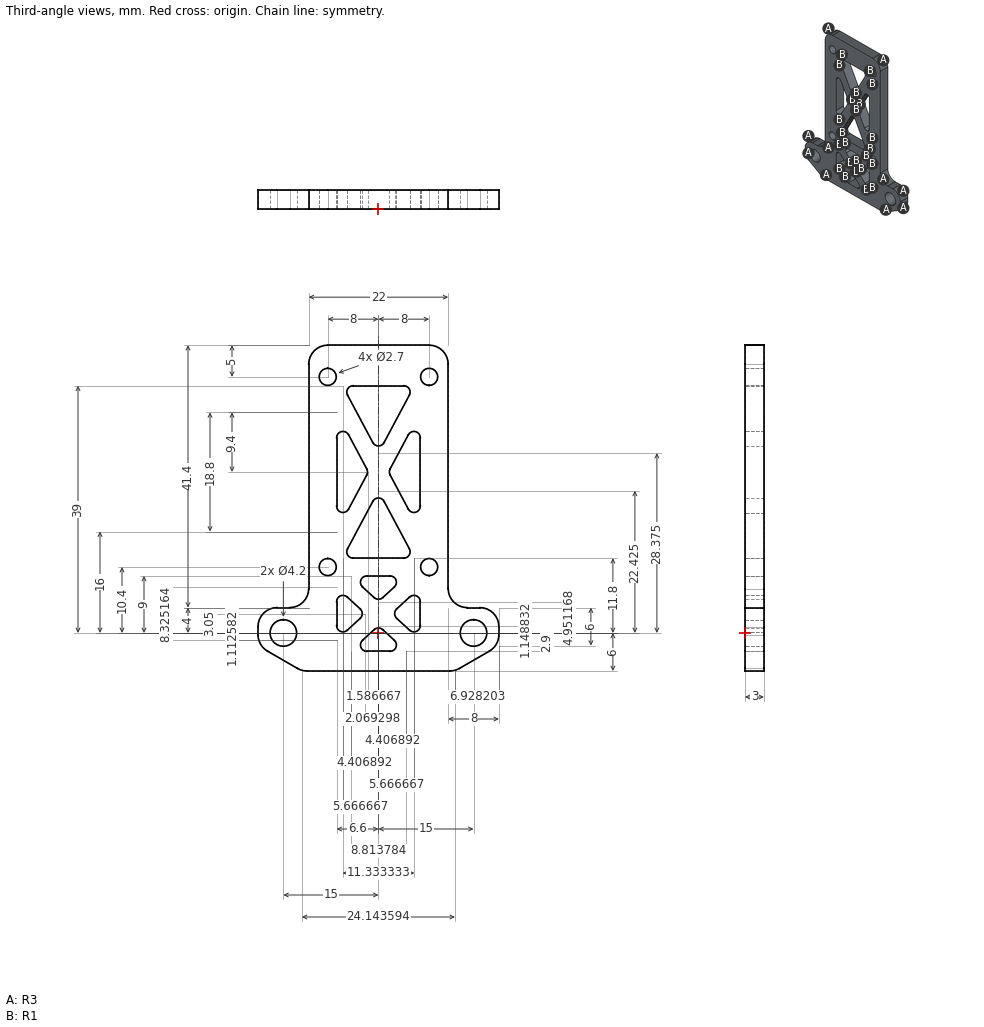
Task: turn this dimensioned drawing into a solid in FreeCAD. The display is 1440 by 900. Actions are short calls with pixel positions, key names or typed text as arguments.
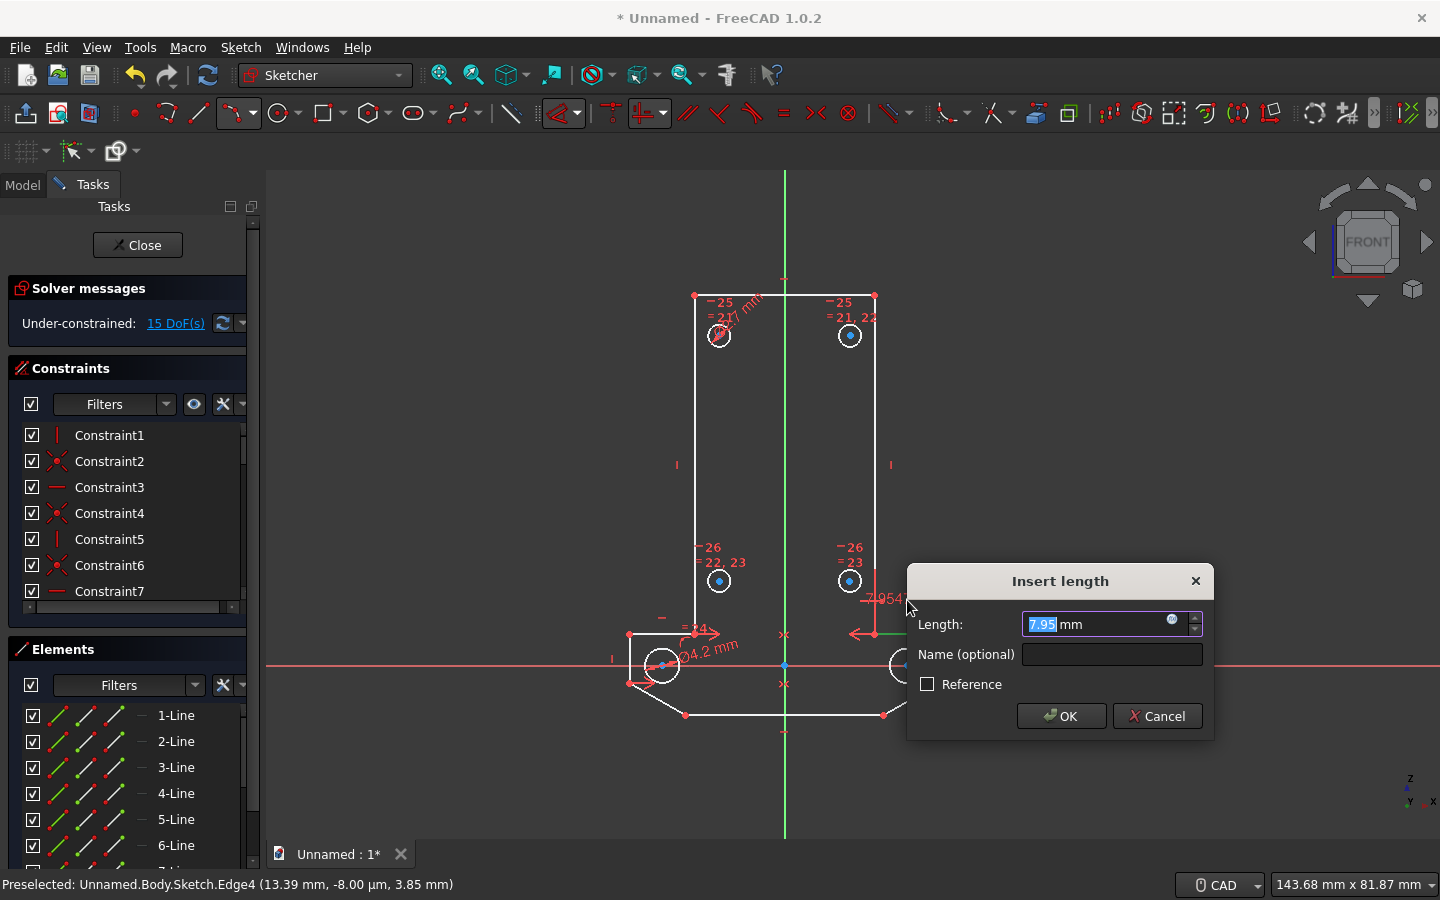
text(8)
key(Return)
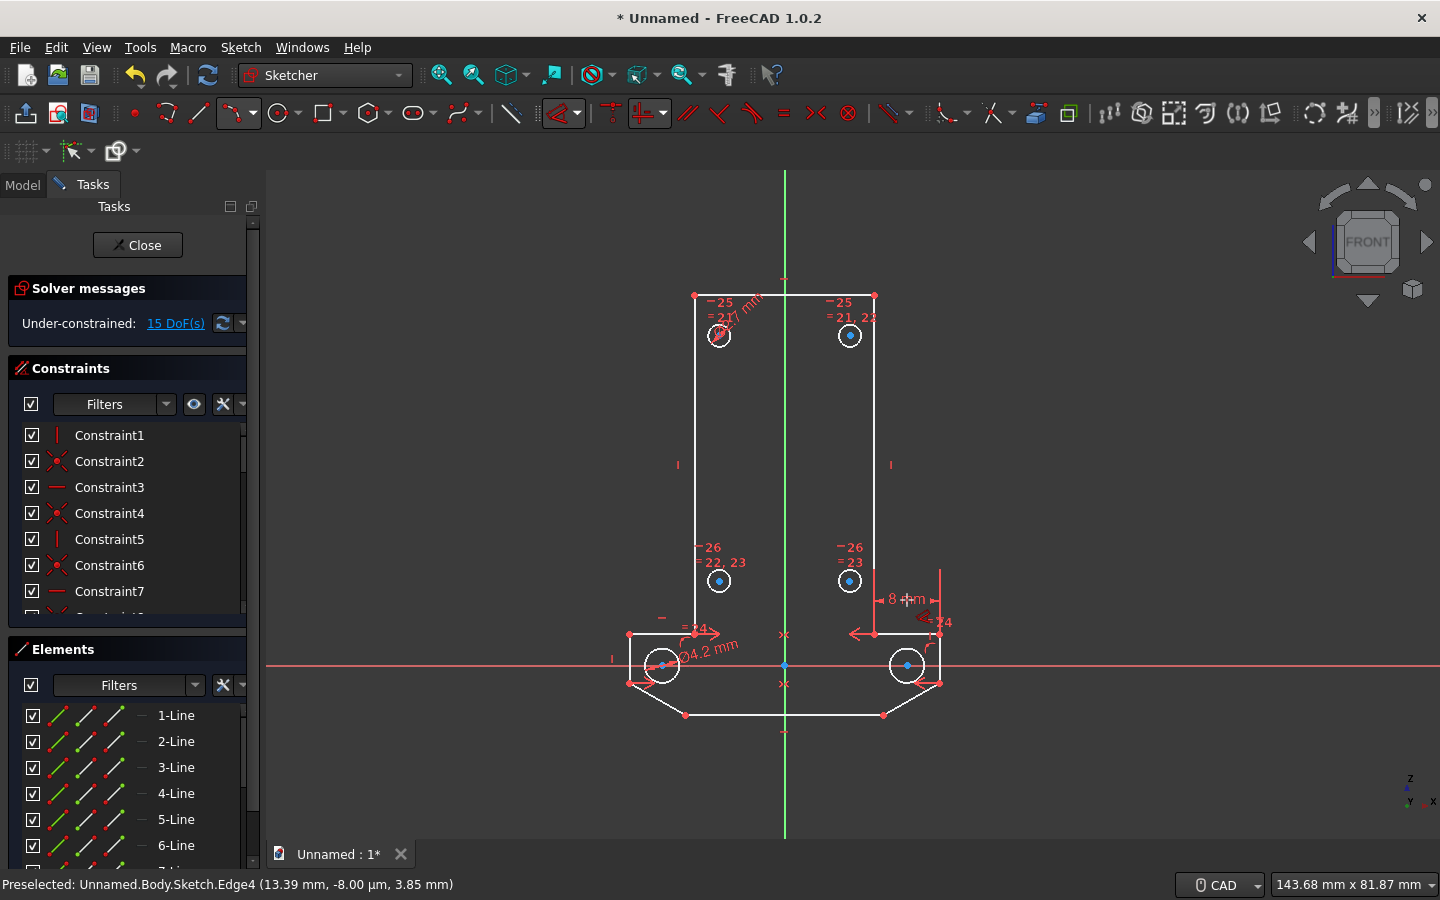
click(940, 649)
click(974, 647)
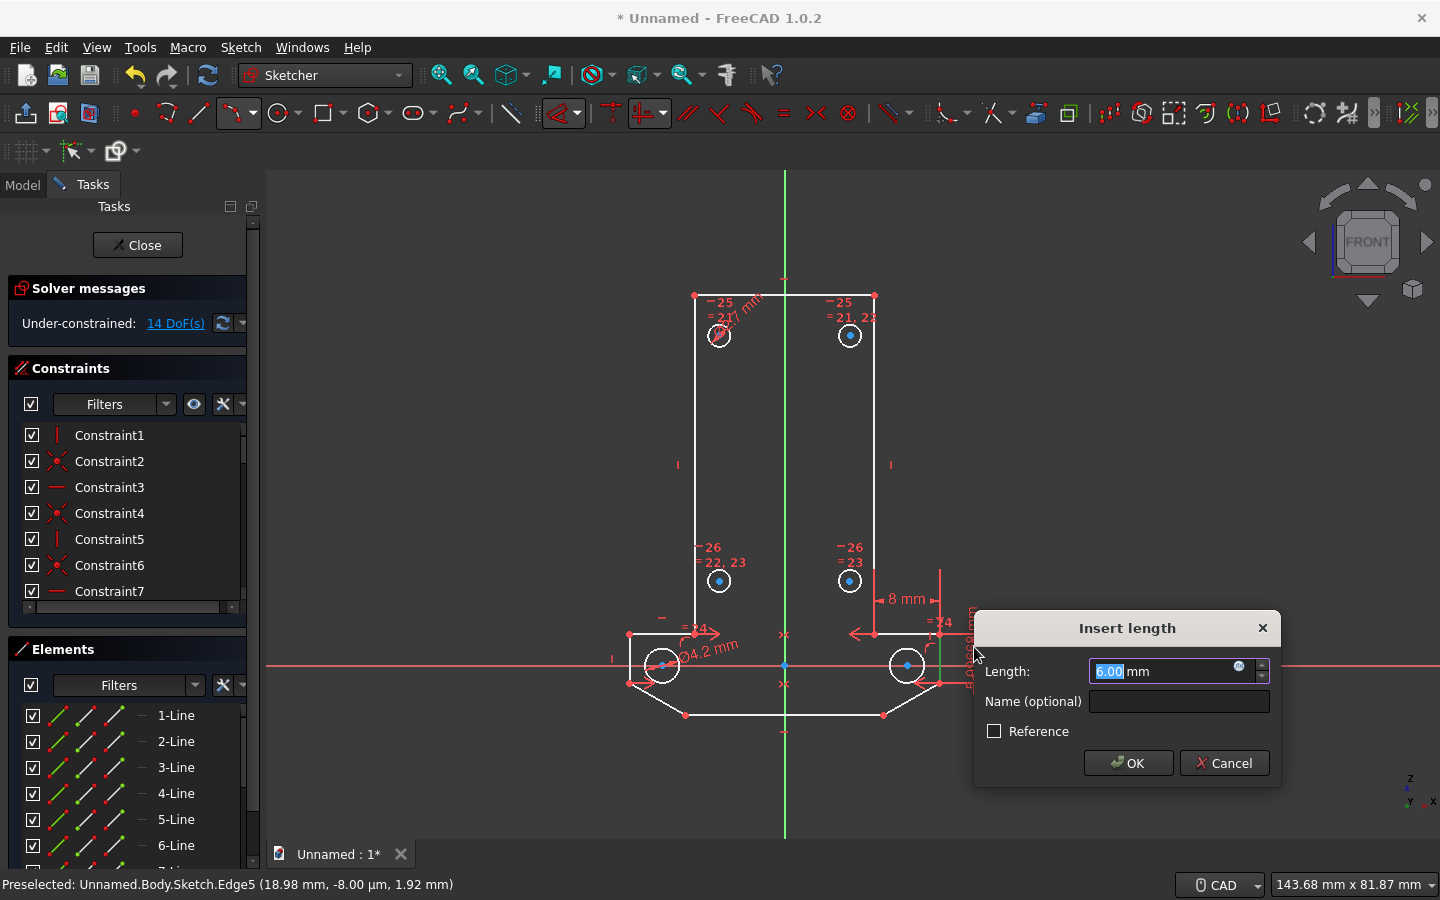
text(6)
key(Return)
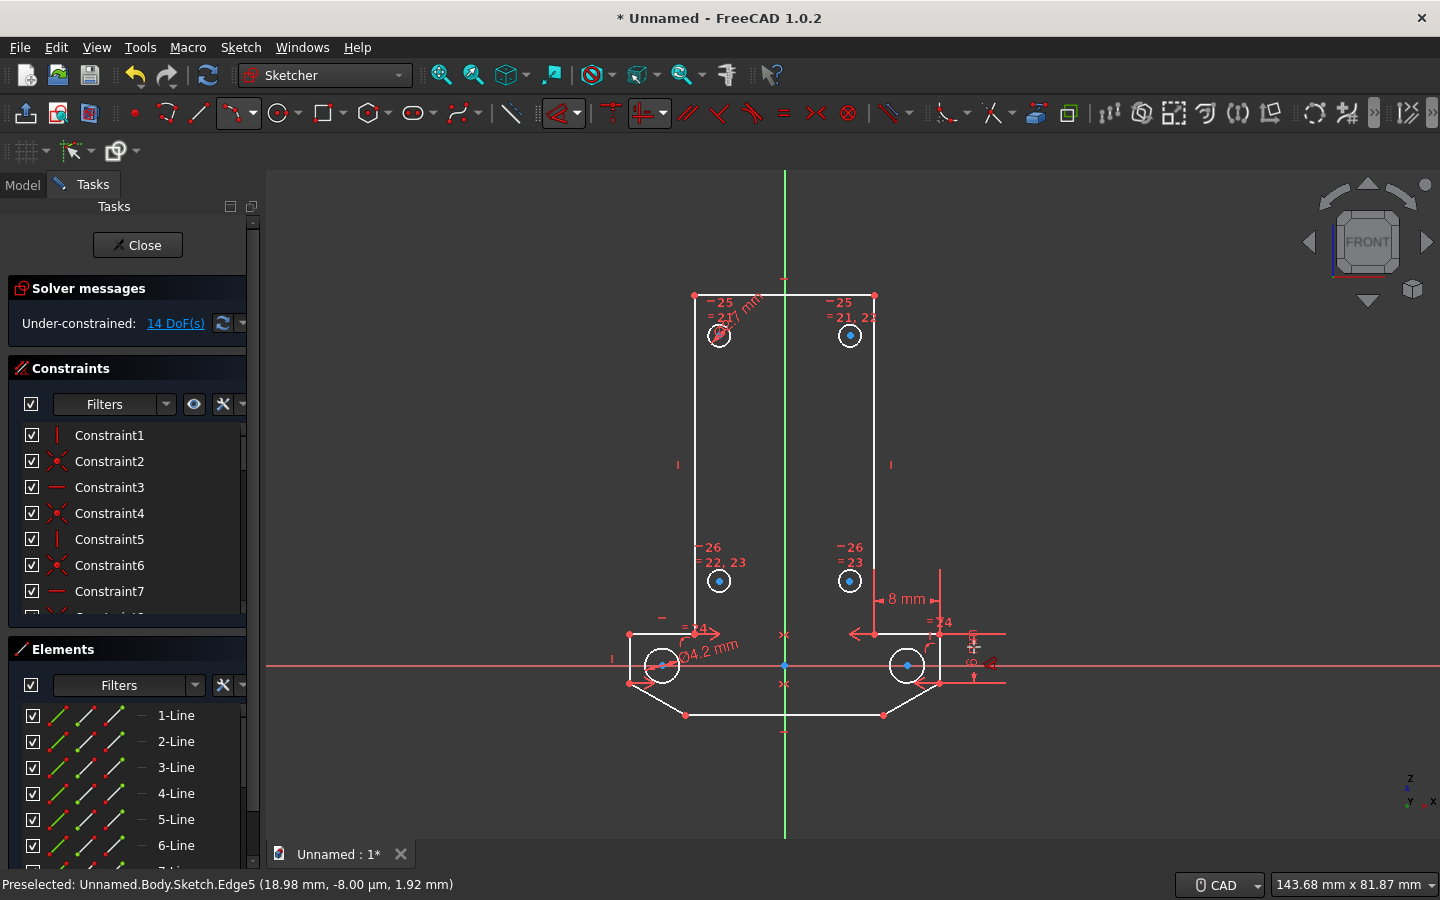
click(719, 336)
click(752, 700)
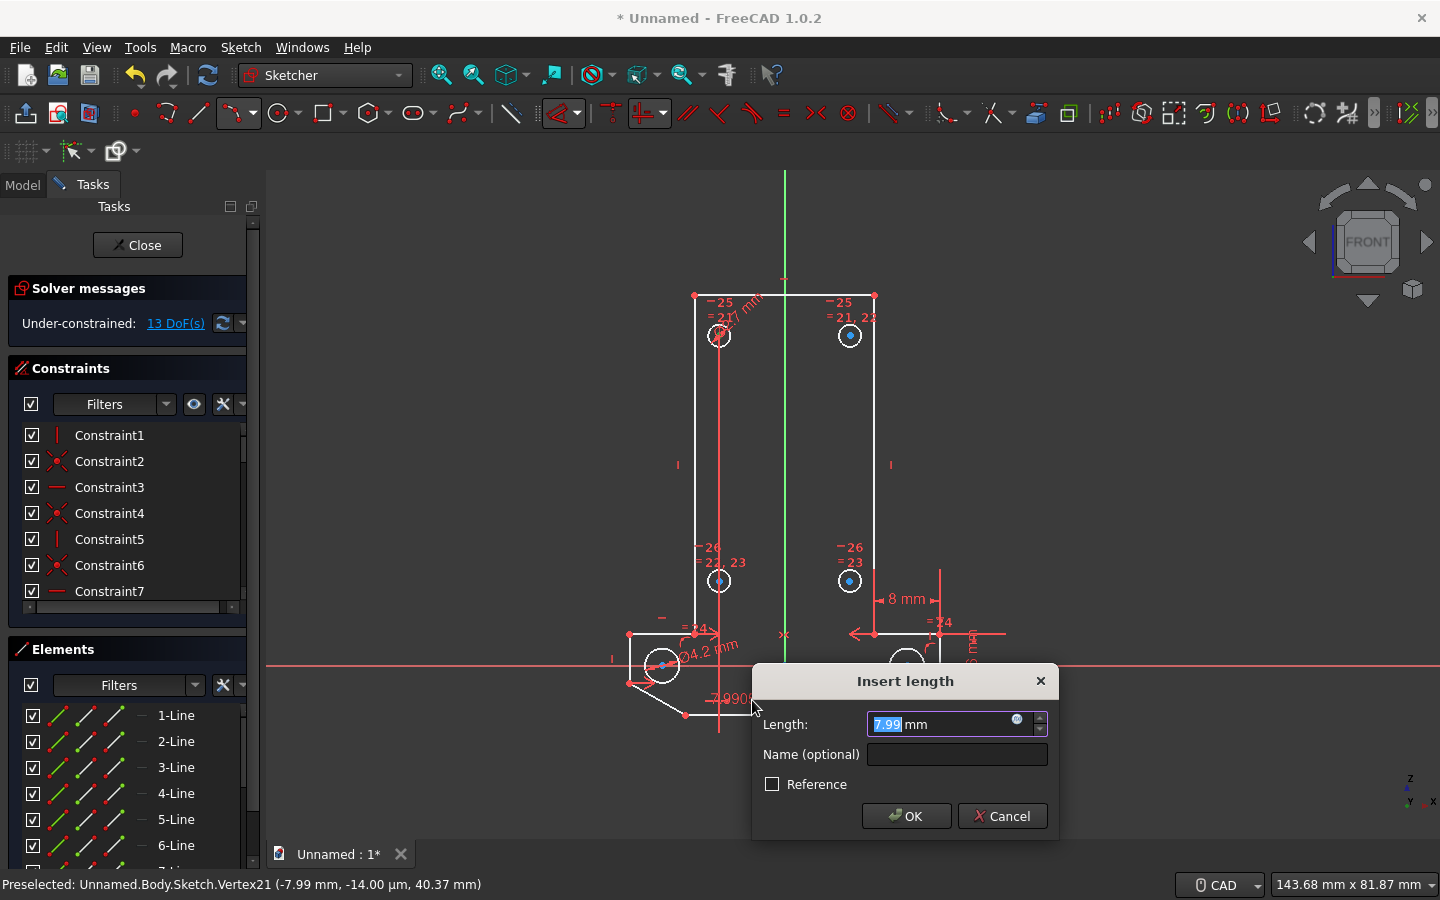
text(8)
key(Return)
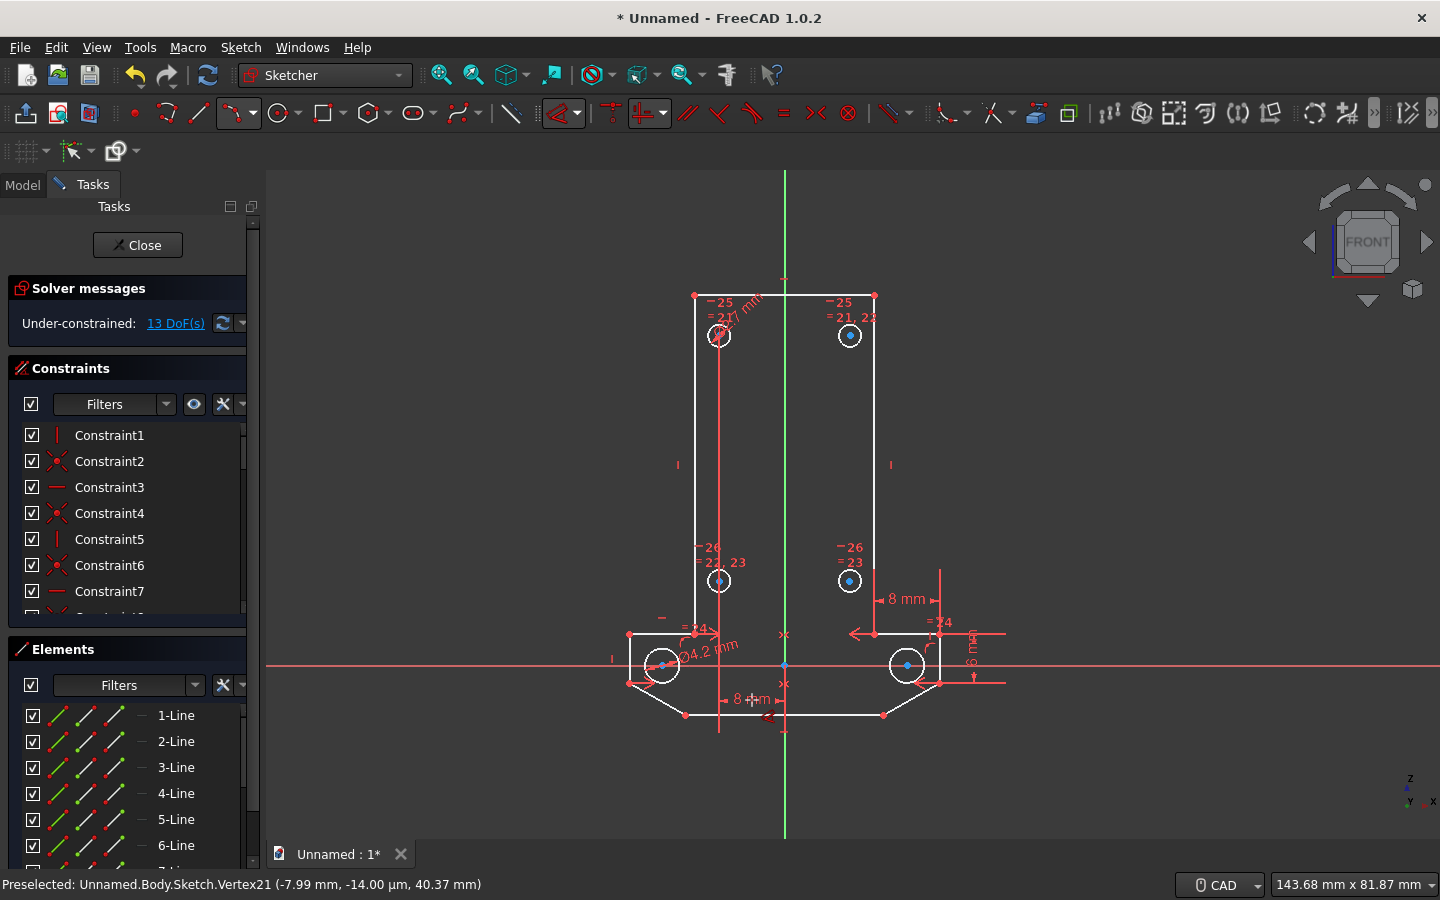
click(850, 336)
click(832, 700)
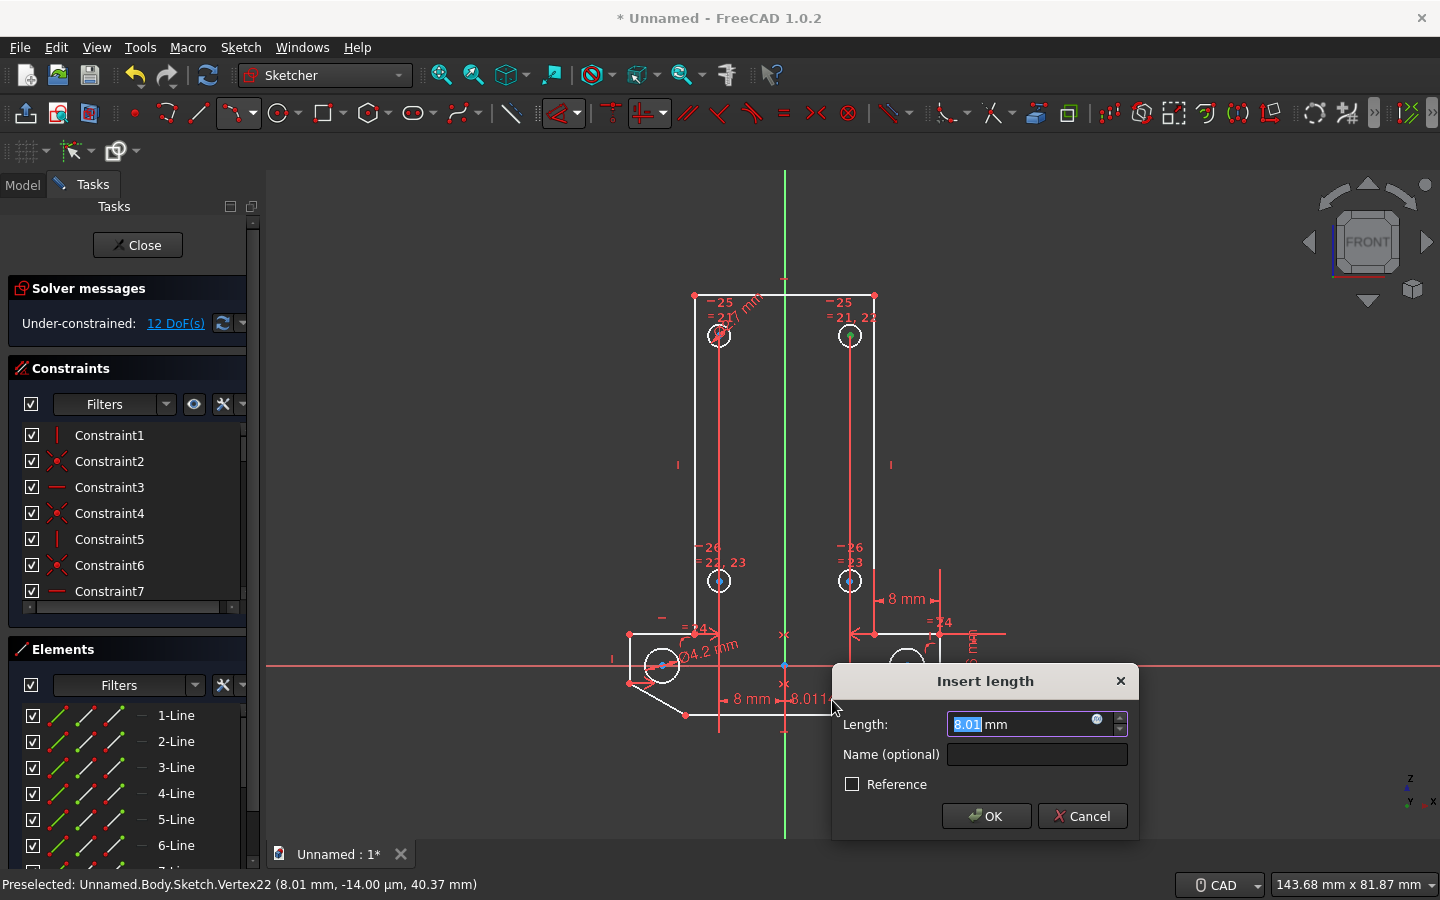
text(8)
key(Return)